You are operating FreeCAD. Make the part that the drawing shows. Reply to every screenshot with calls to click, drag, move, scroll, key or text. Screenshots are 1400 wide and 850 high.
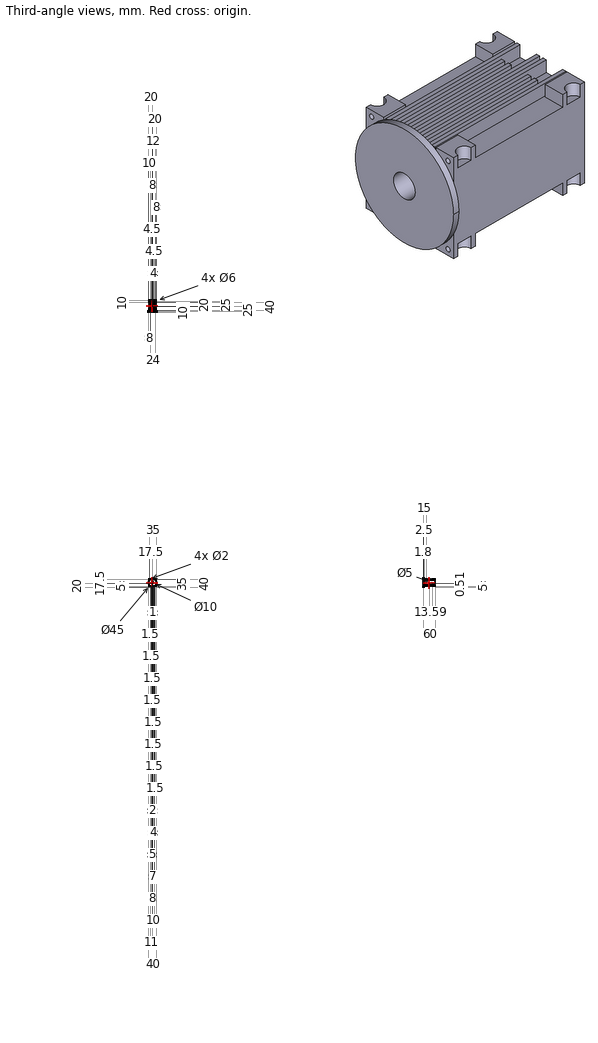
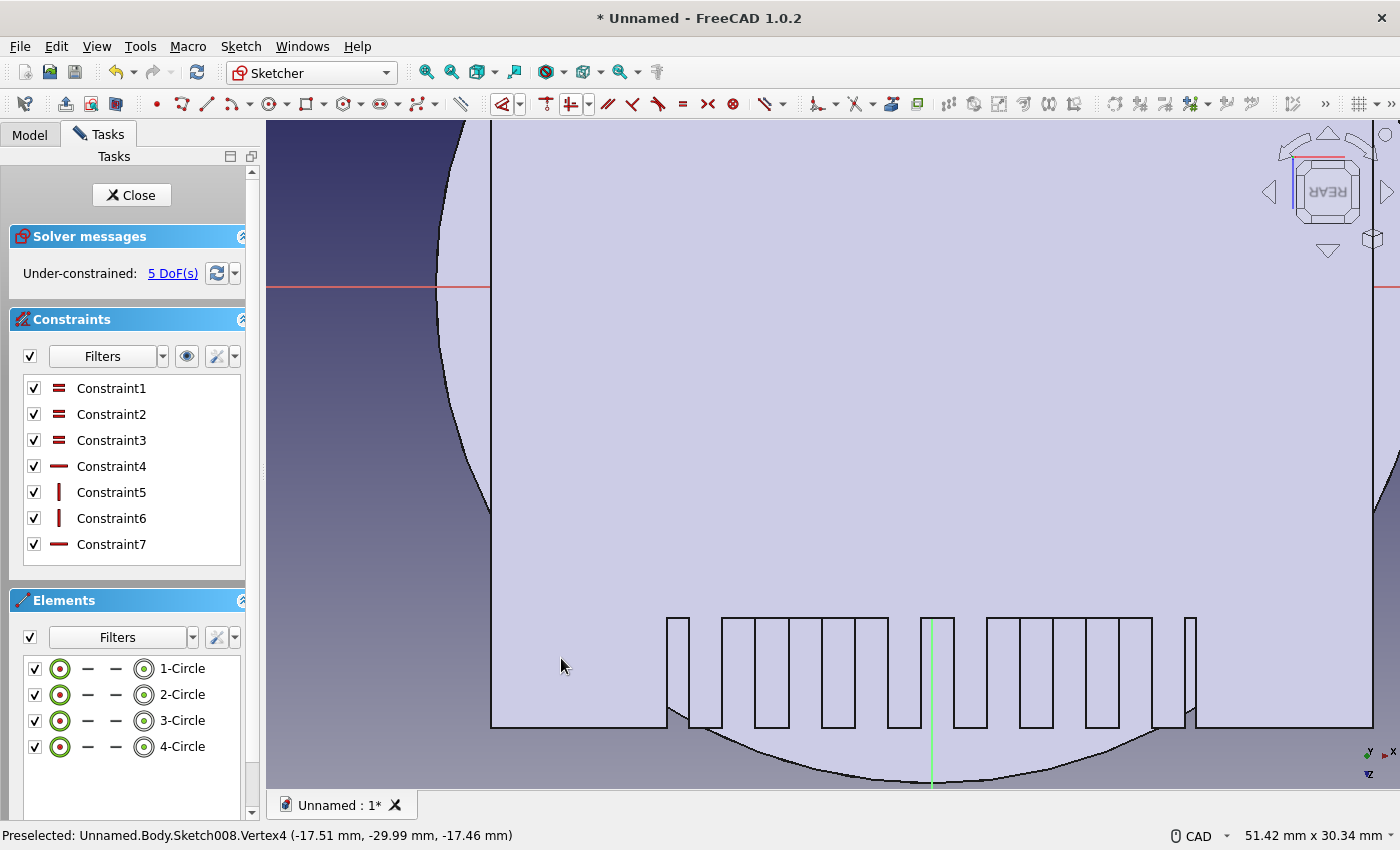
click(561, 658)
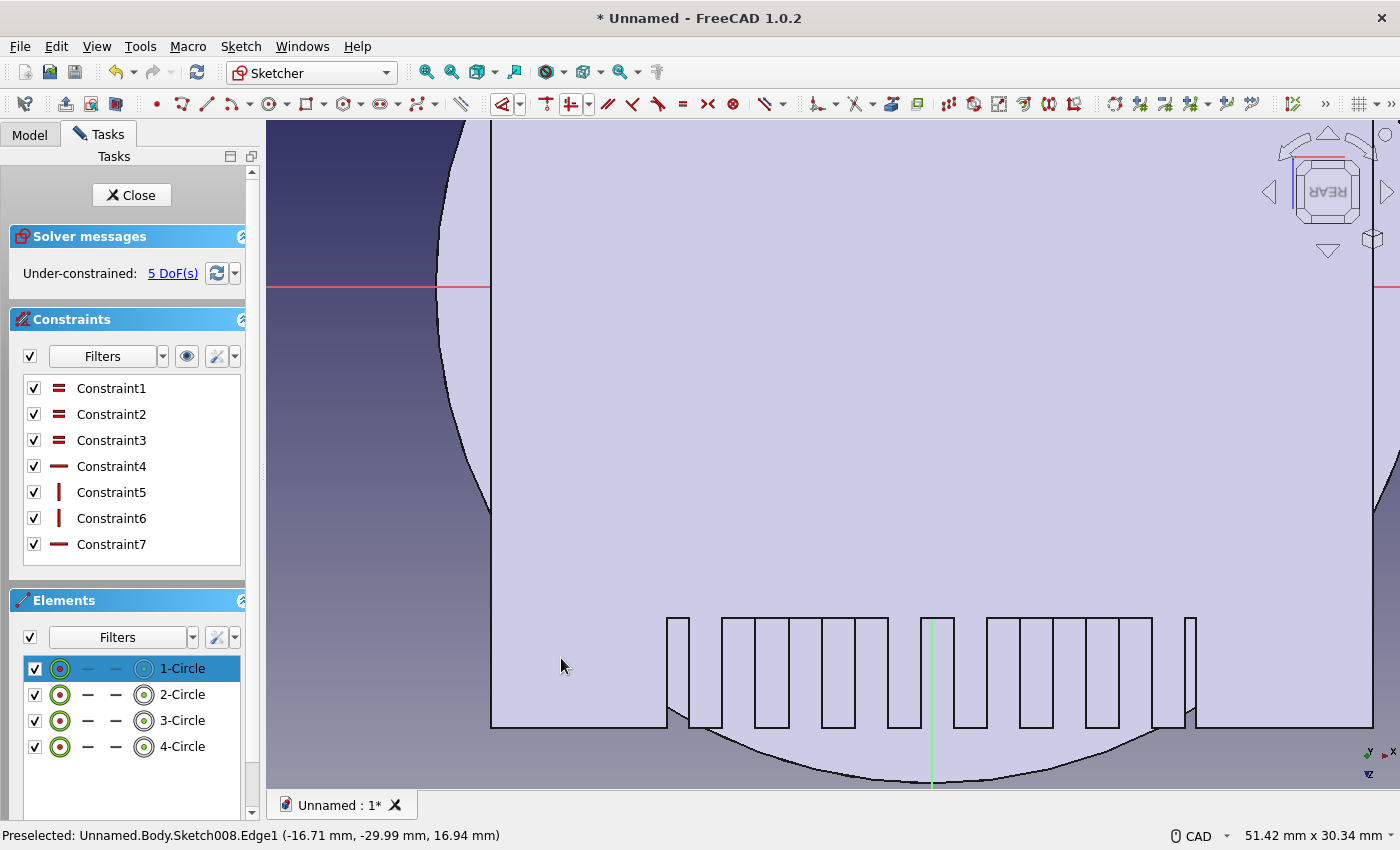
click(520, 104)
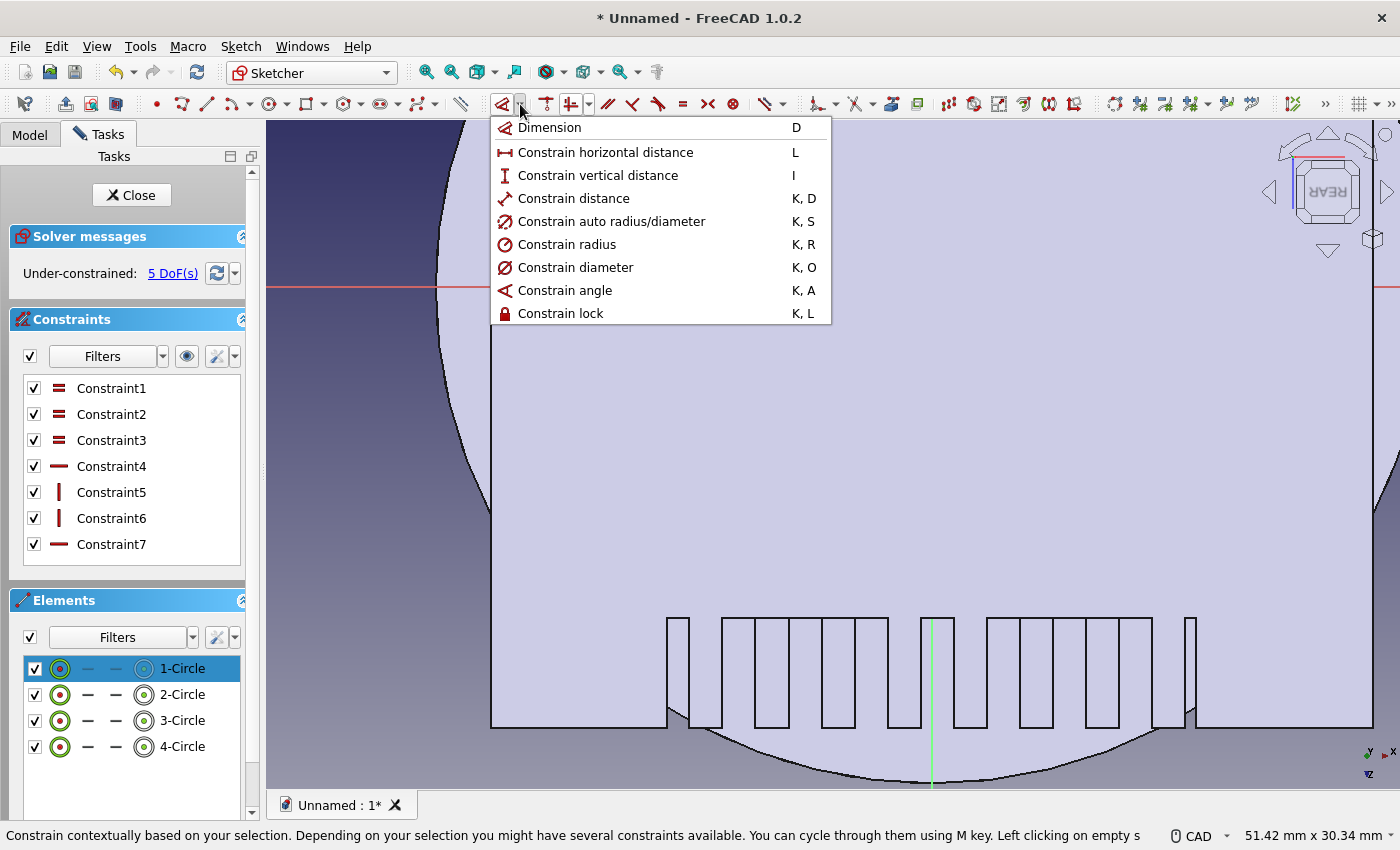
click(661, 268)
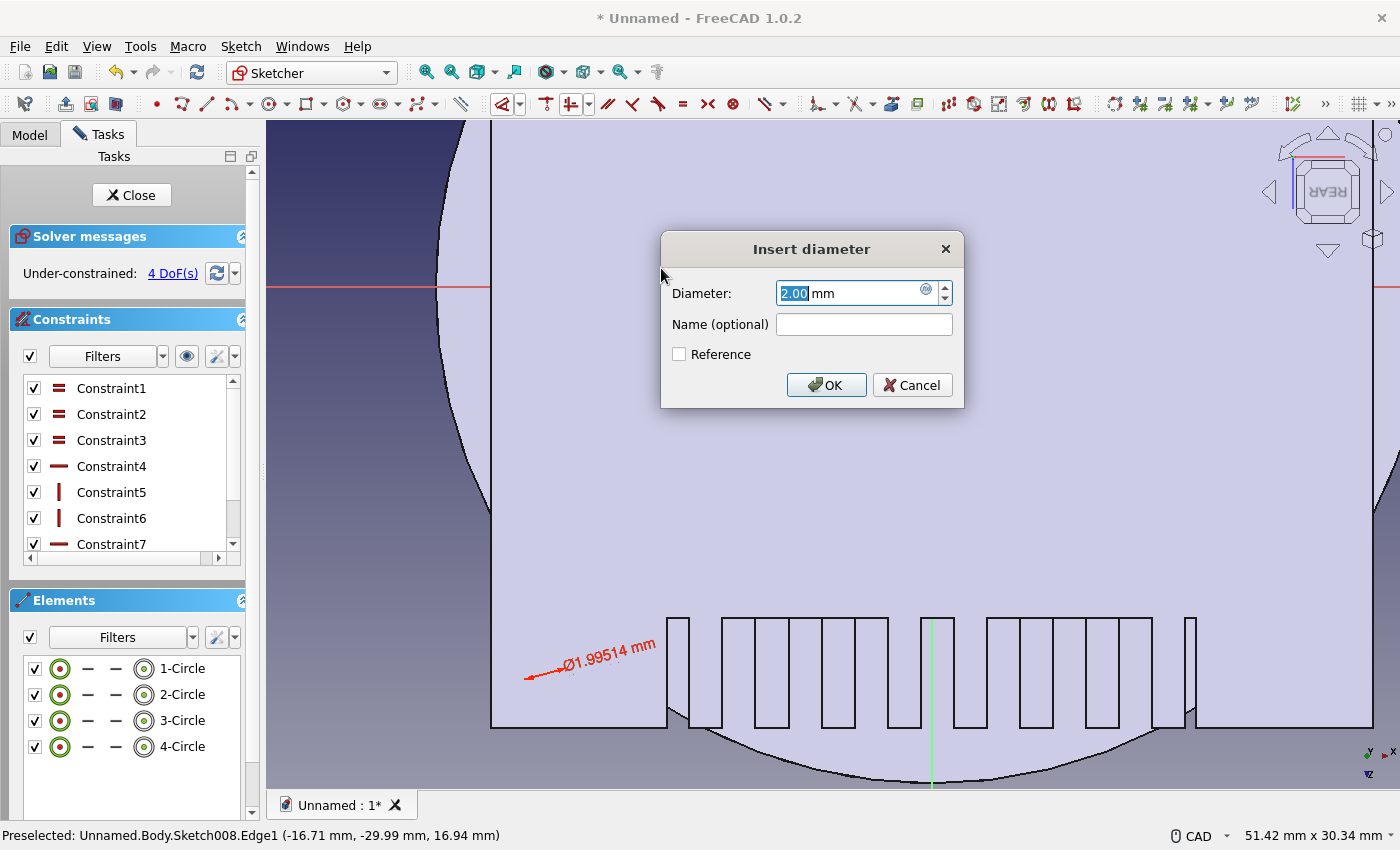
text(2)
key(Return)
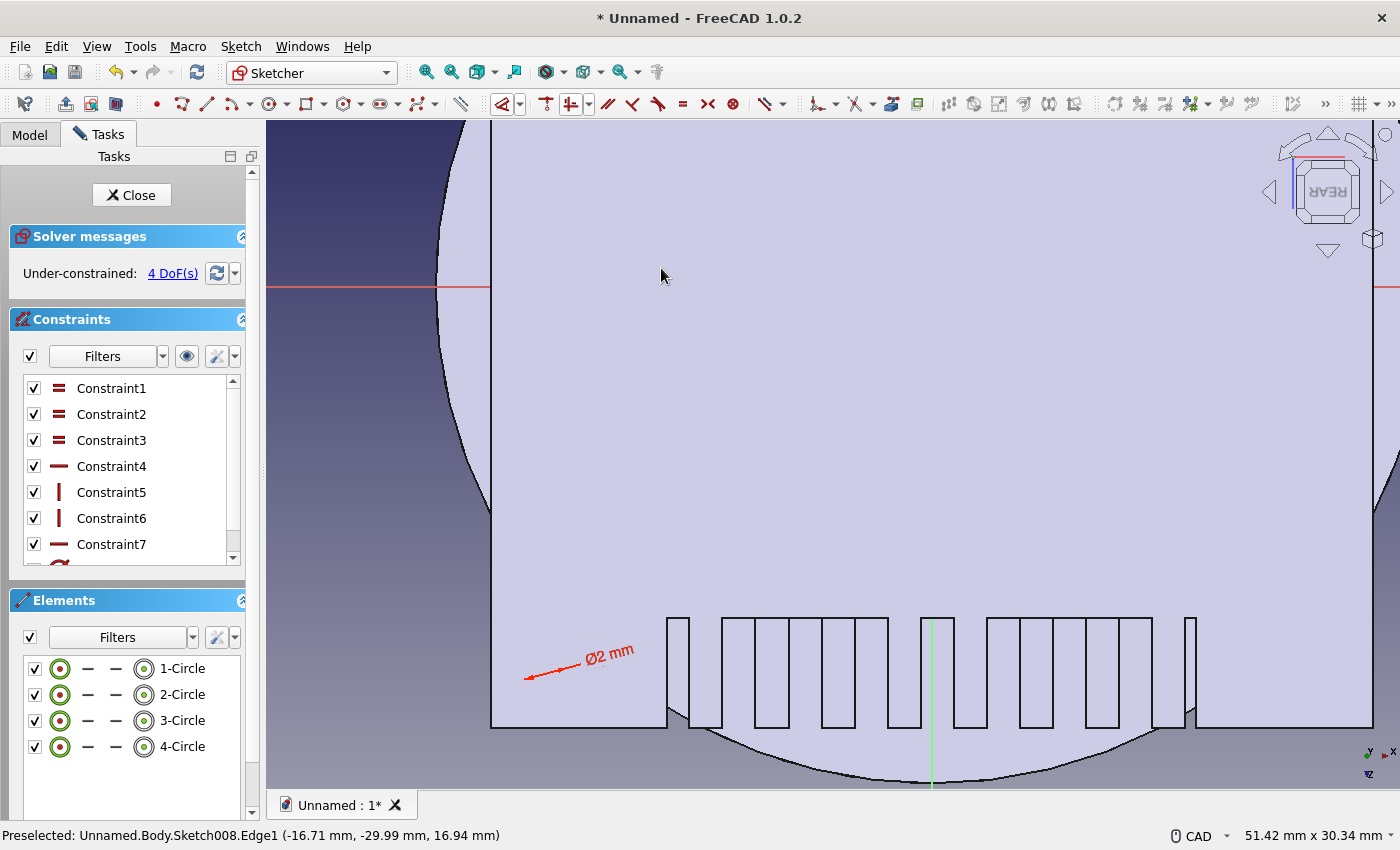
click(546, 674)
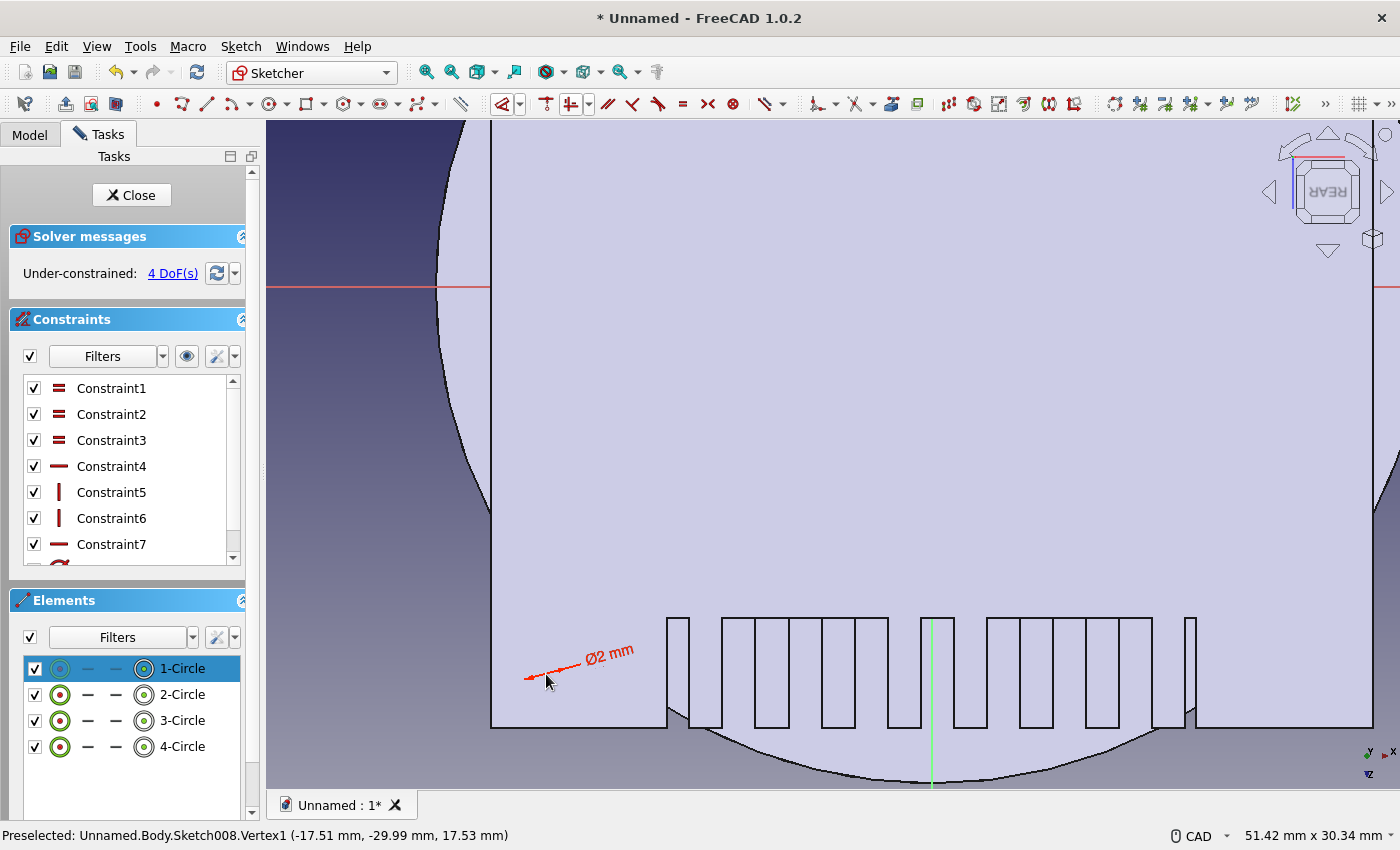
scroll(561, 658, down, 3)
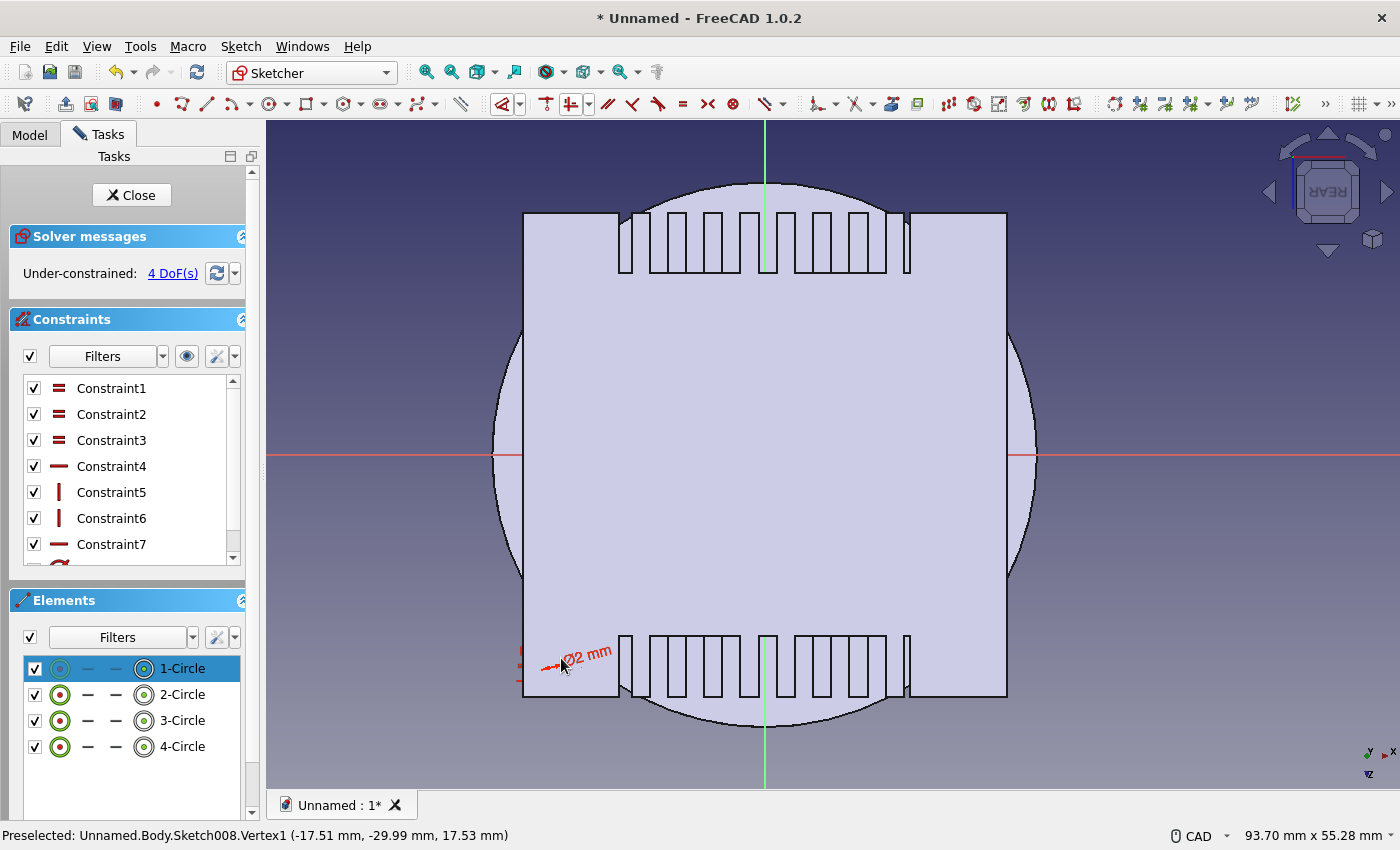
click(976, 667)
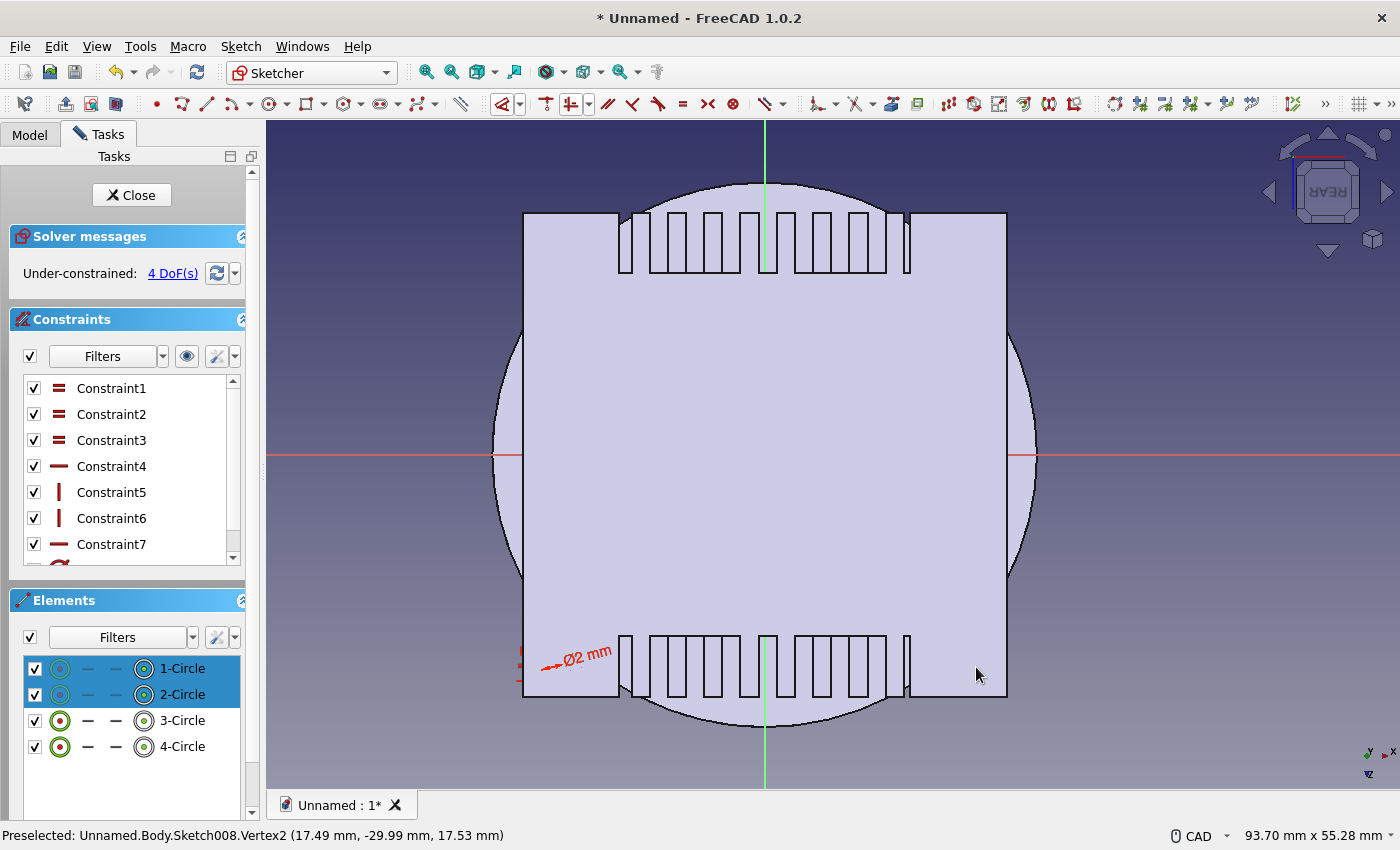
key(l)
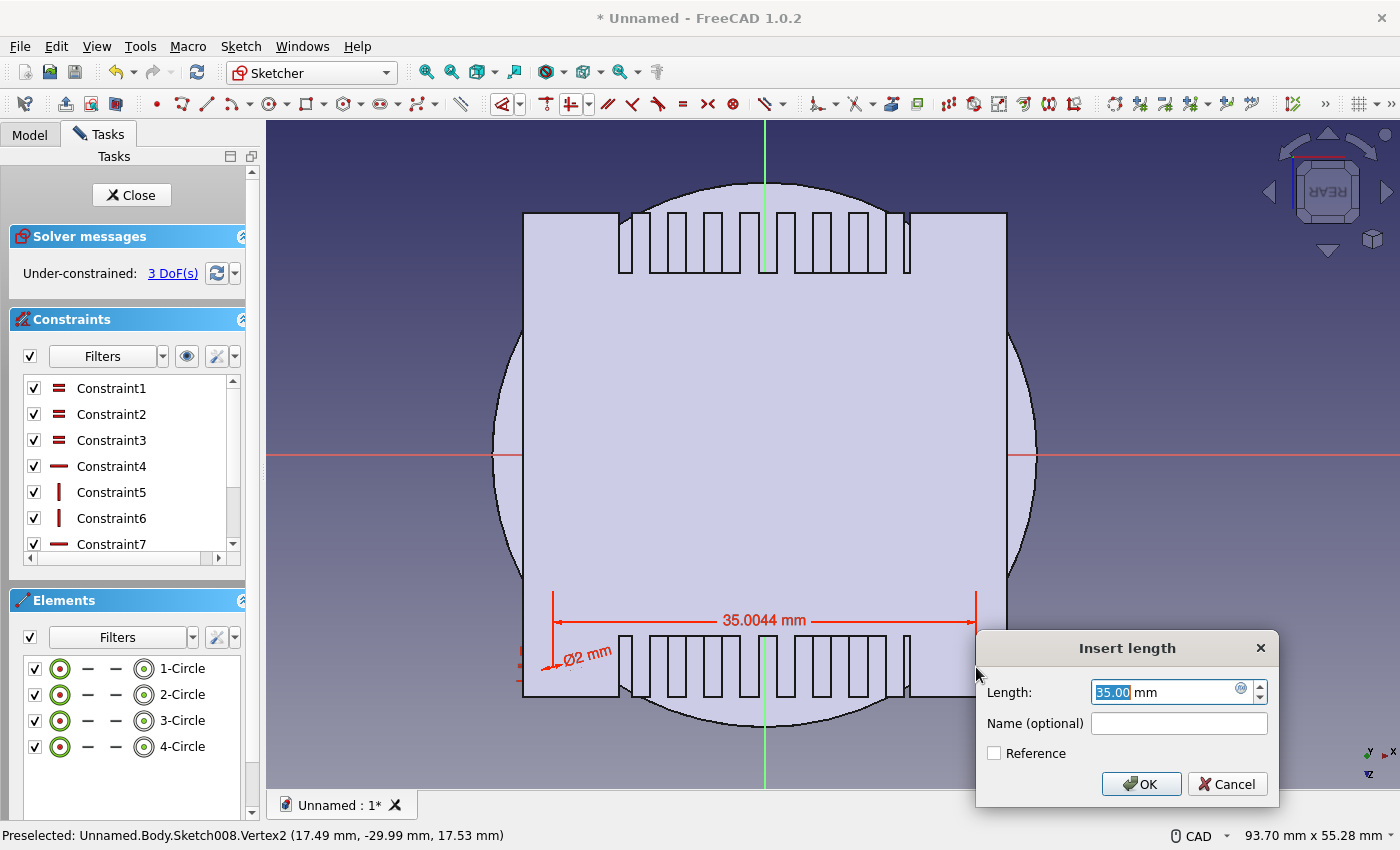
text(35)
key(Return)